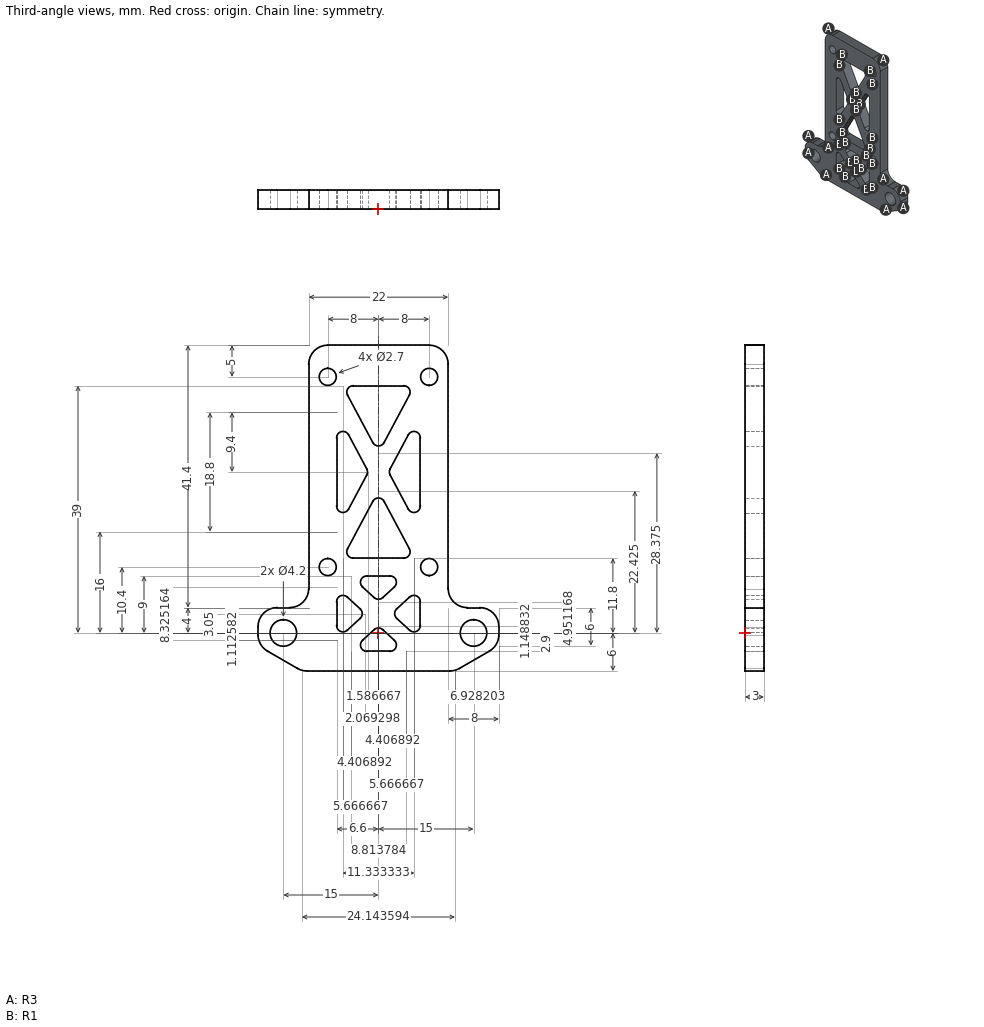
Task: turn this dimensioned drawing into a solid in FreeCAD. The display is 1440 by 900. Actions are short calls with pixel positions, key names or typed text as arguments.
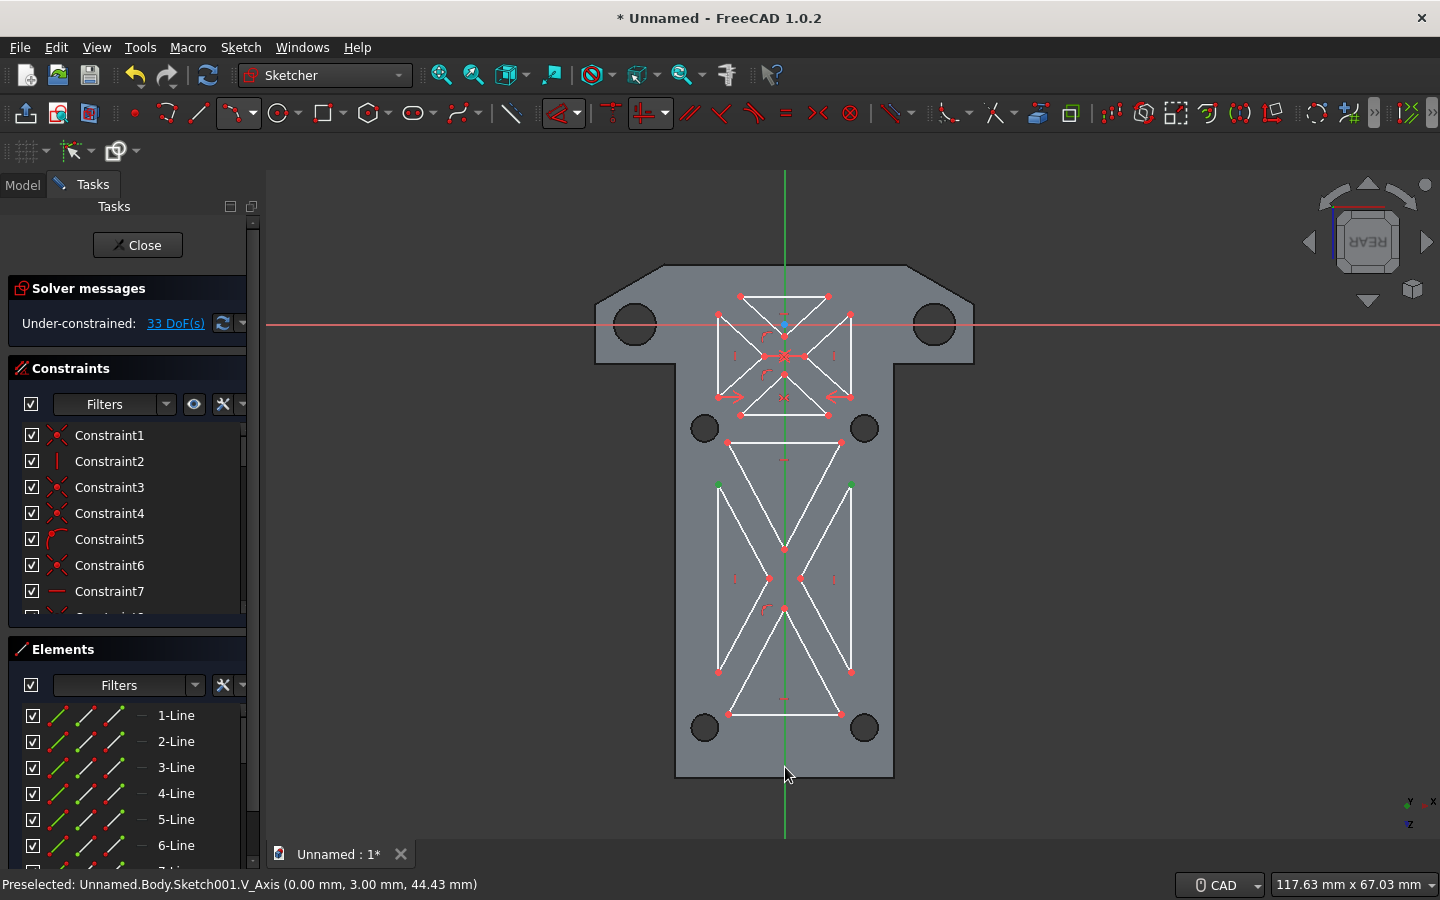
click(818, 114)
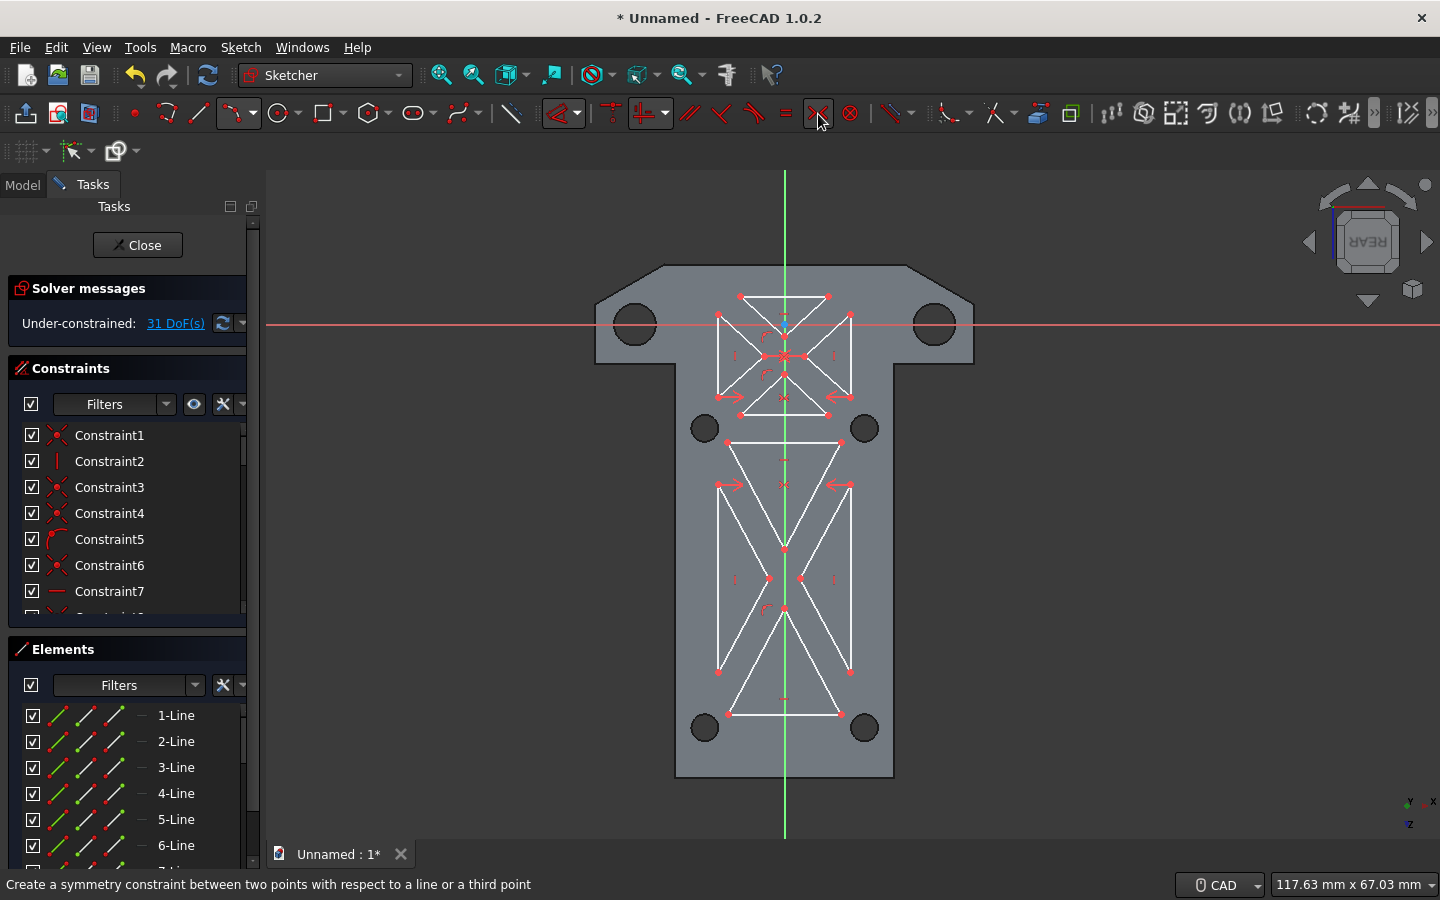
click(769, 579)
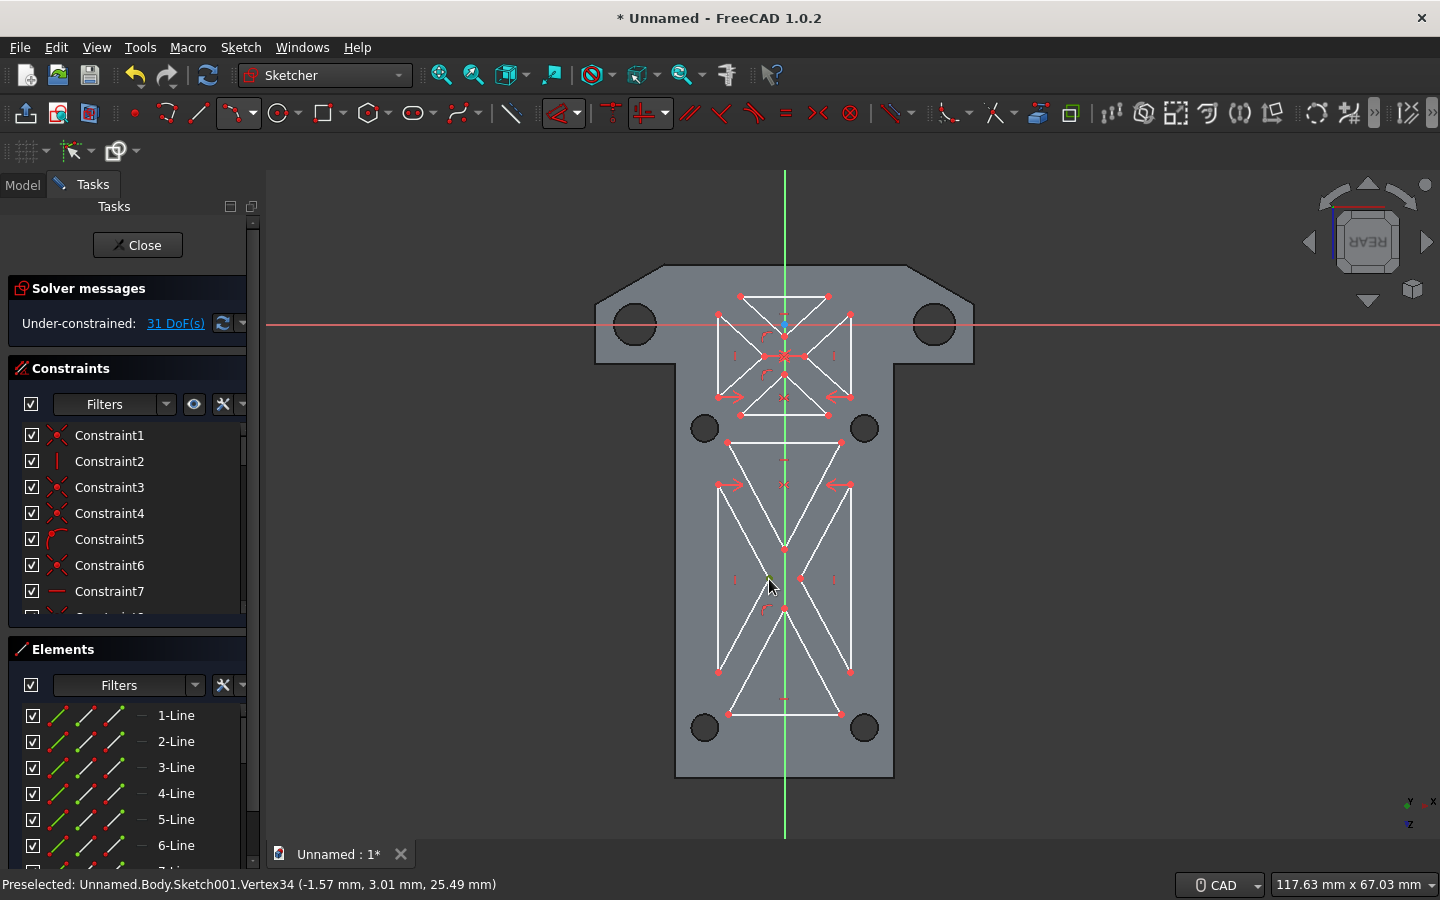
click(800, 579)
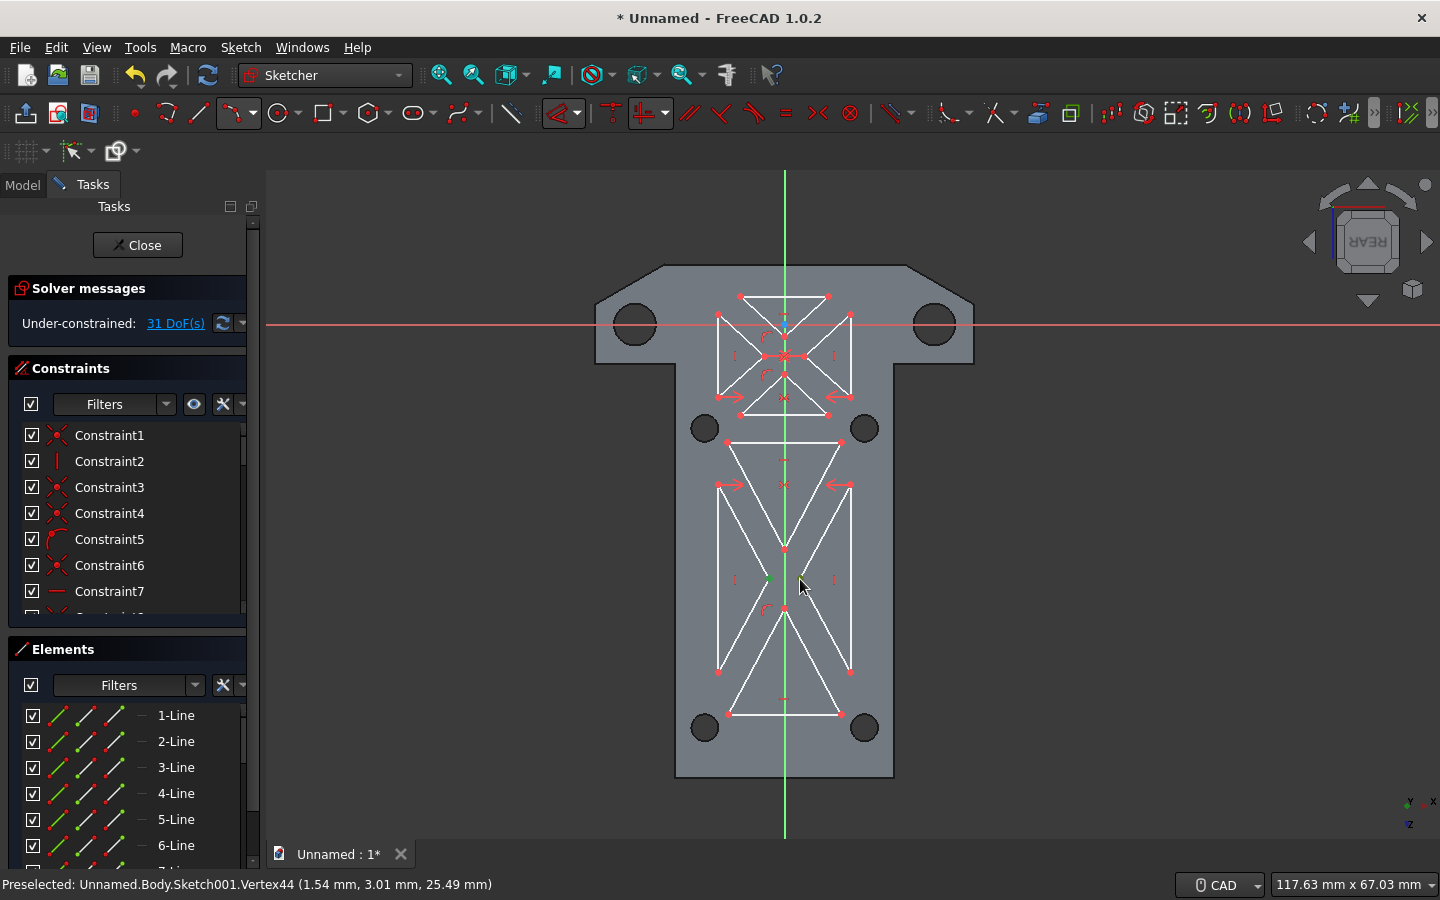
click(785, 767)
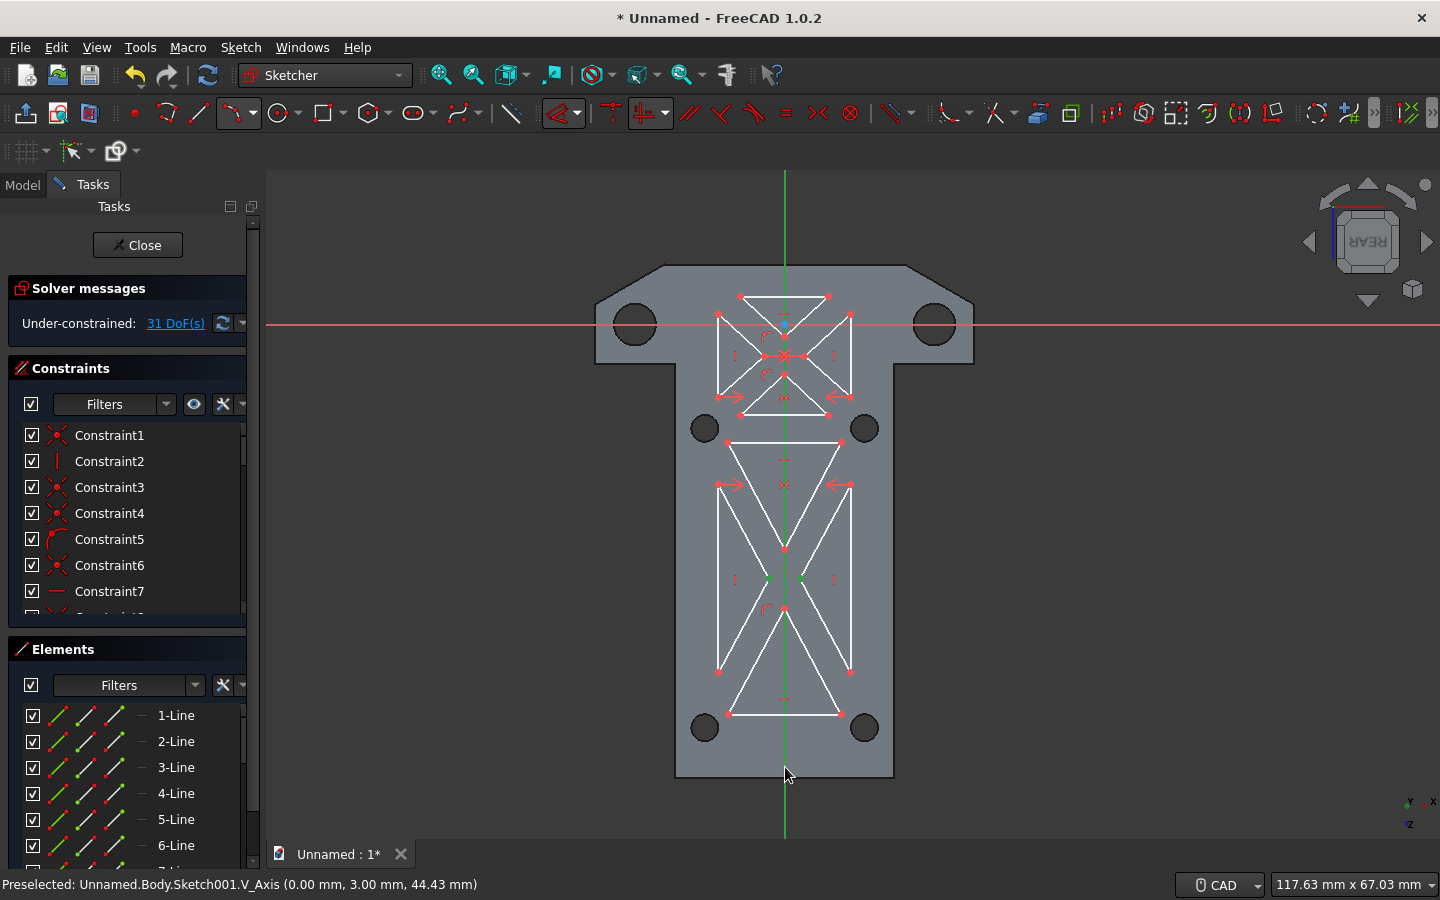
click(818, 114)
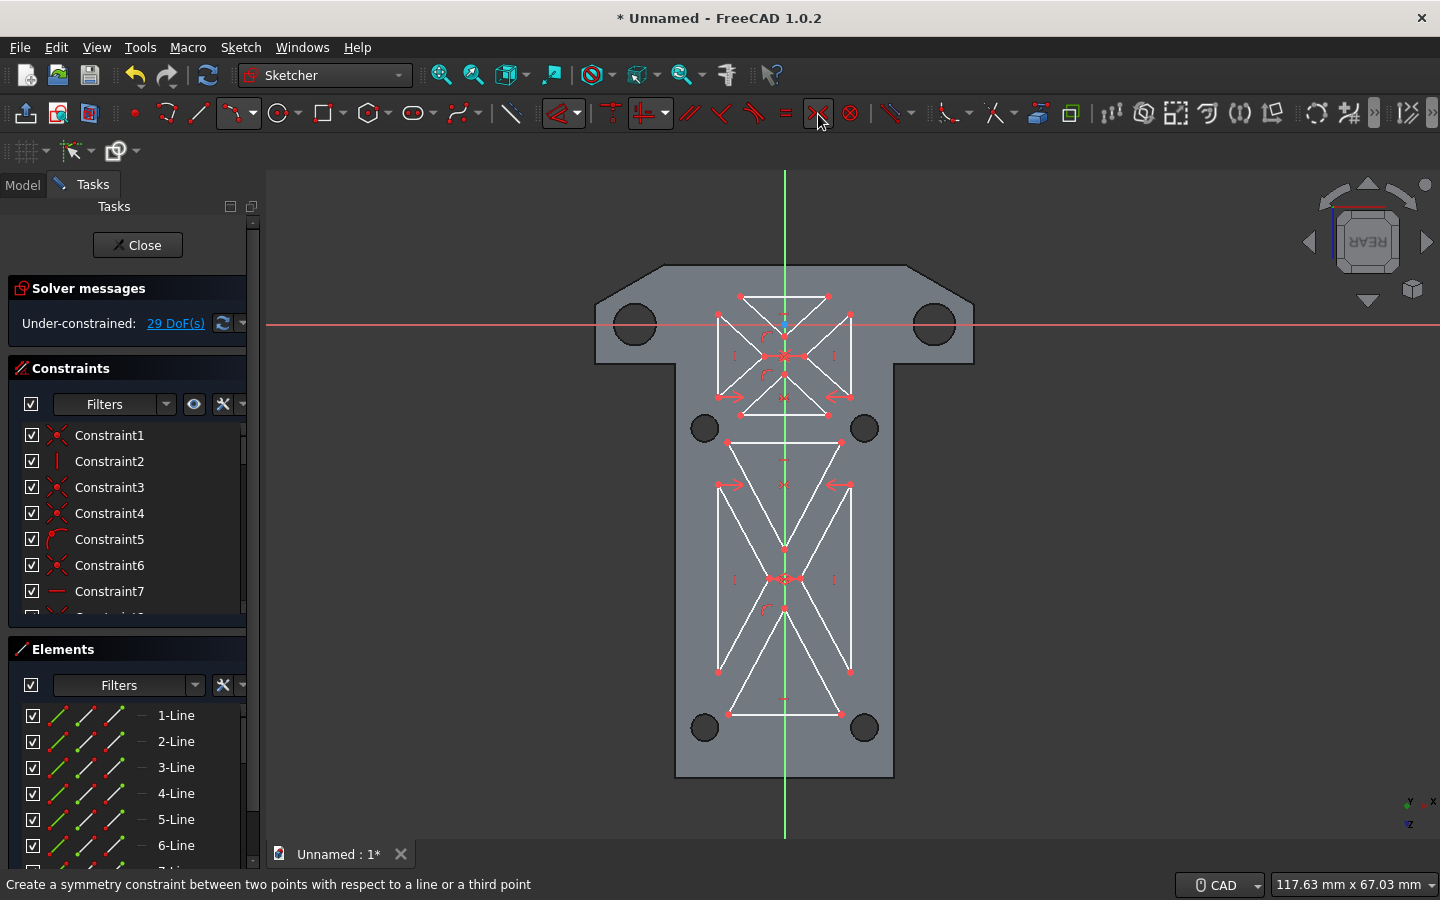
click(785, 549)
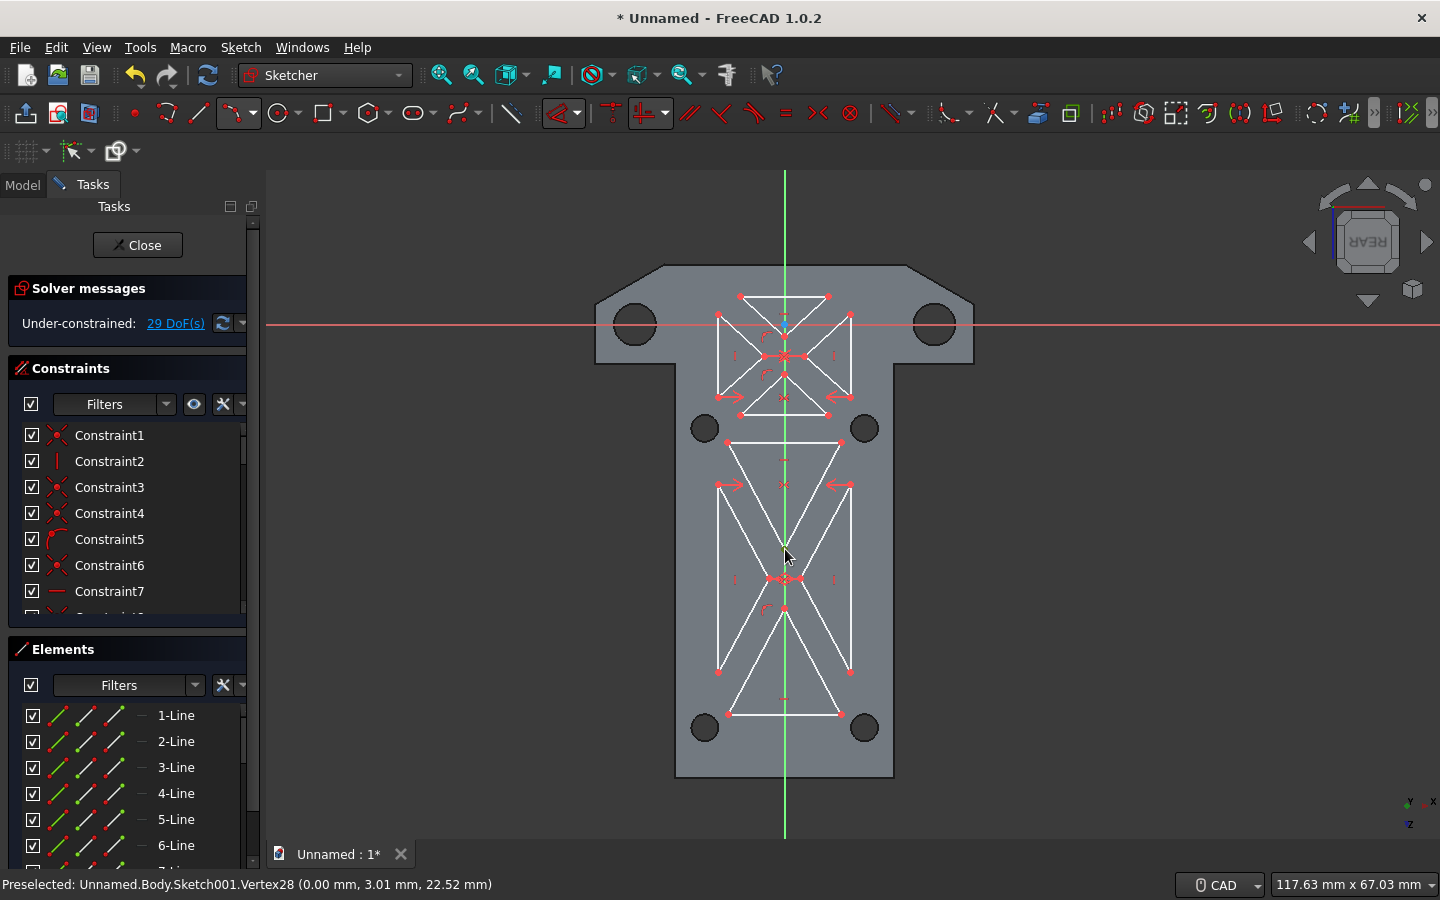
click(785, 767)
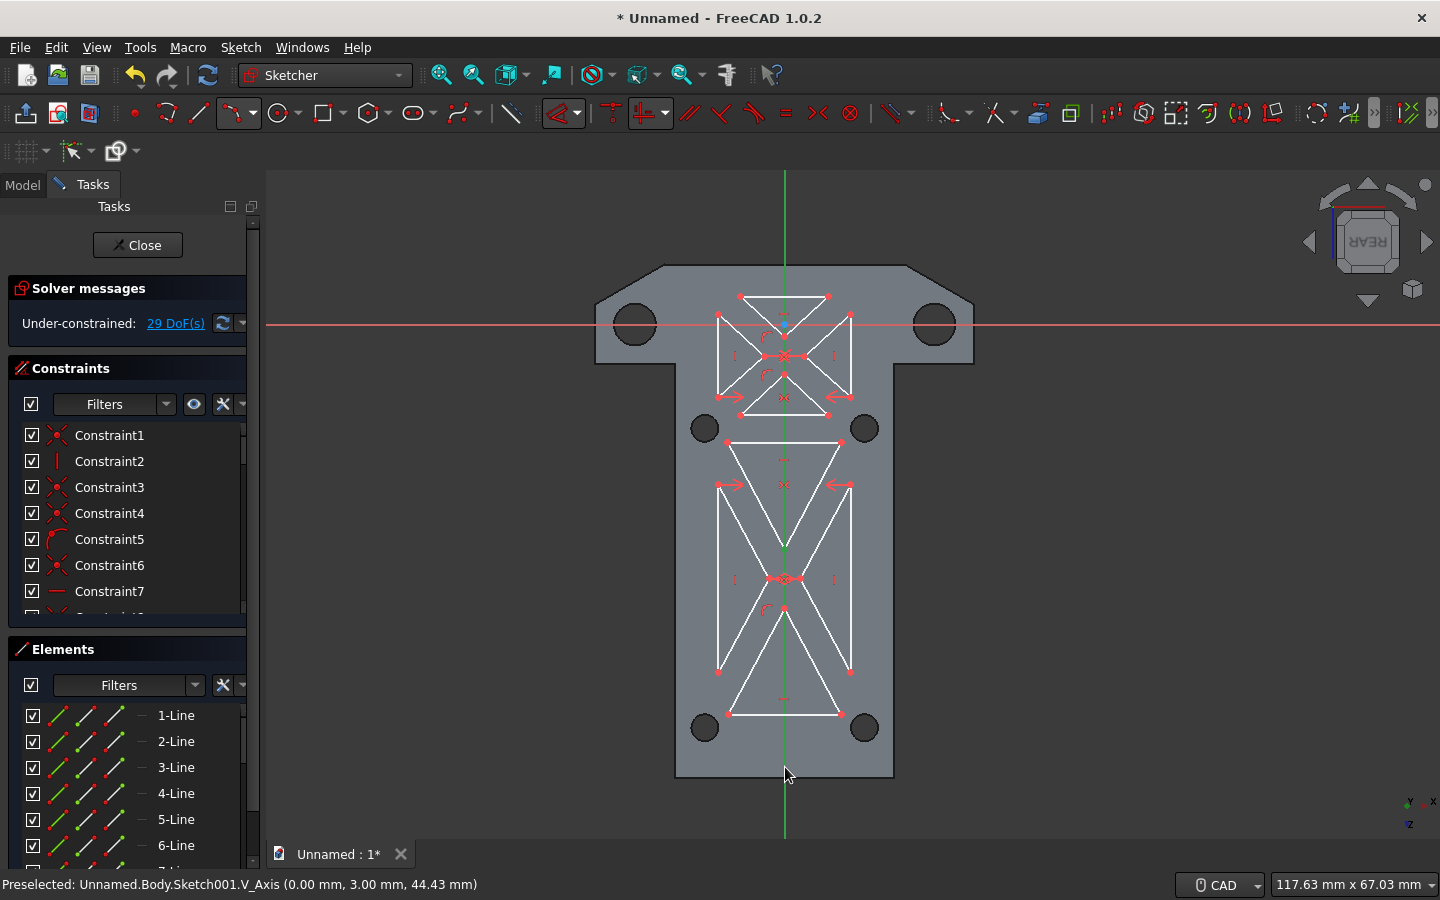
key(c)